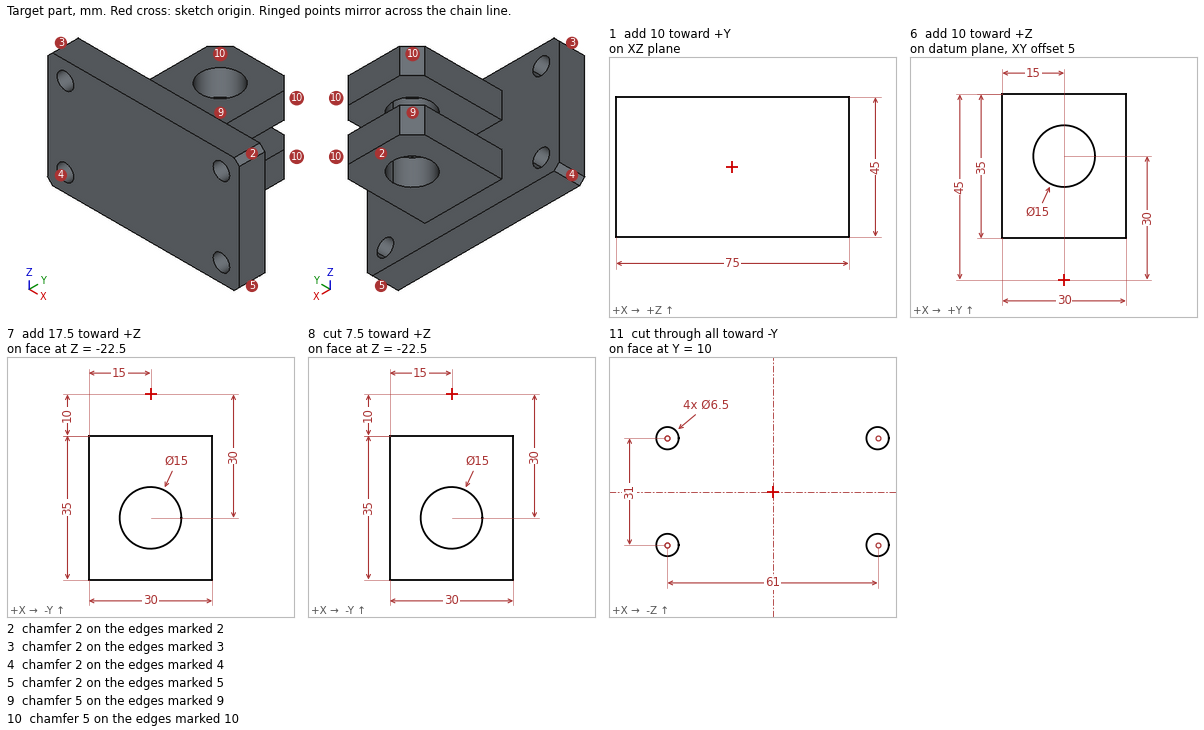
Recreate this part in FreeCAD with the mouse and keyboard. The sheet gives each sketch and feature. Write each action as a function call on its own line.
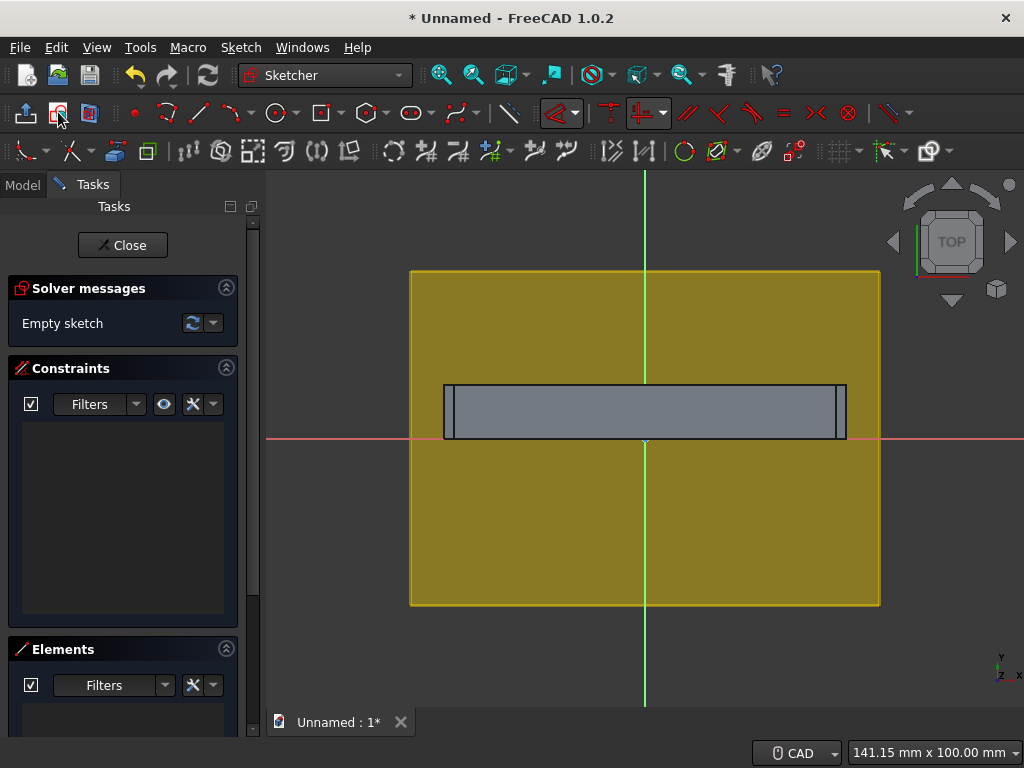
key(q)
key(s)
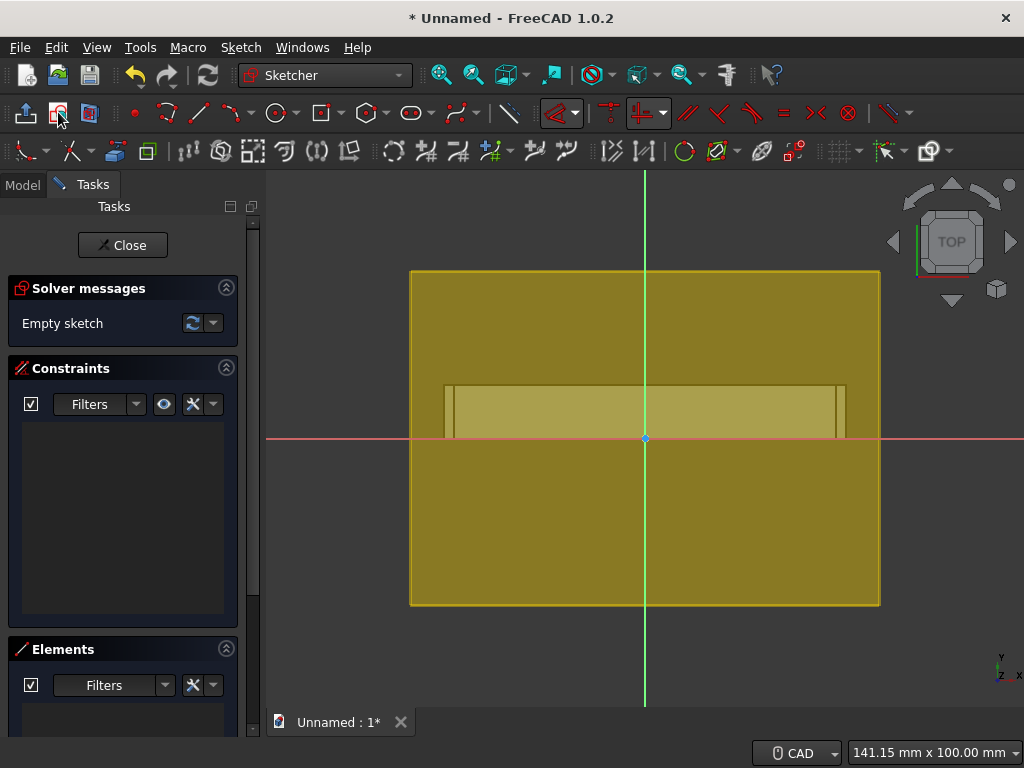
scroll(294, 679, down, 1)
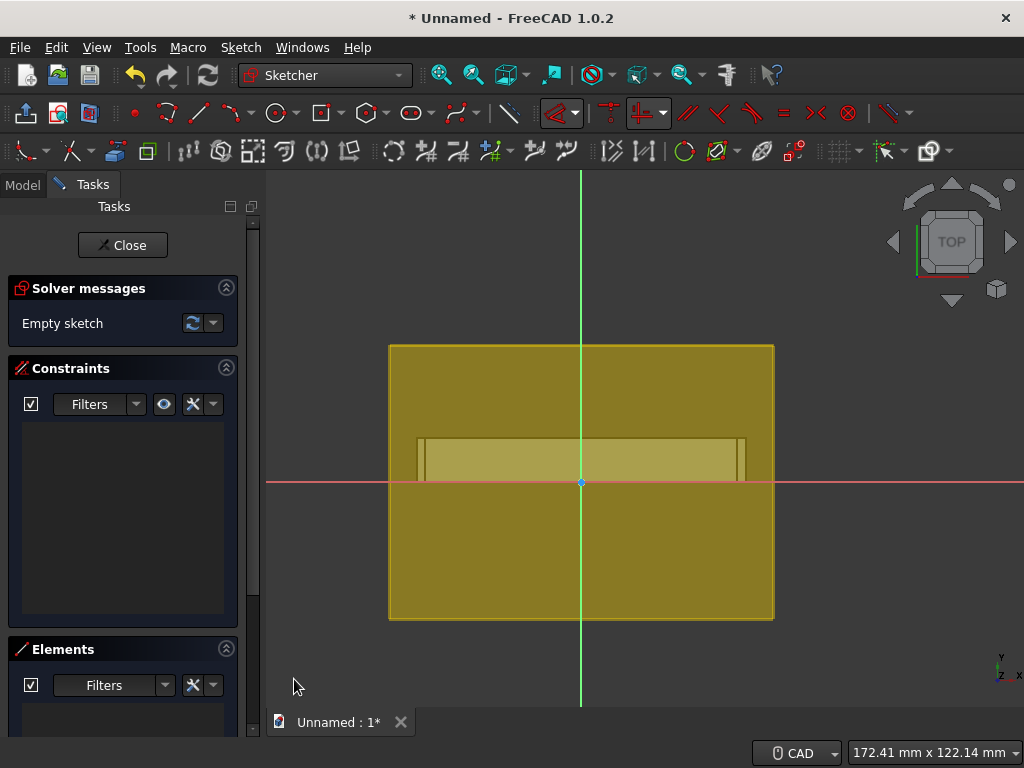
scroll(587, 316, up, 3)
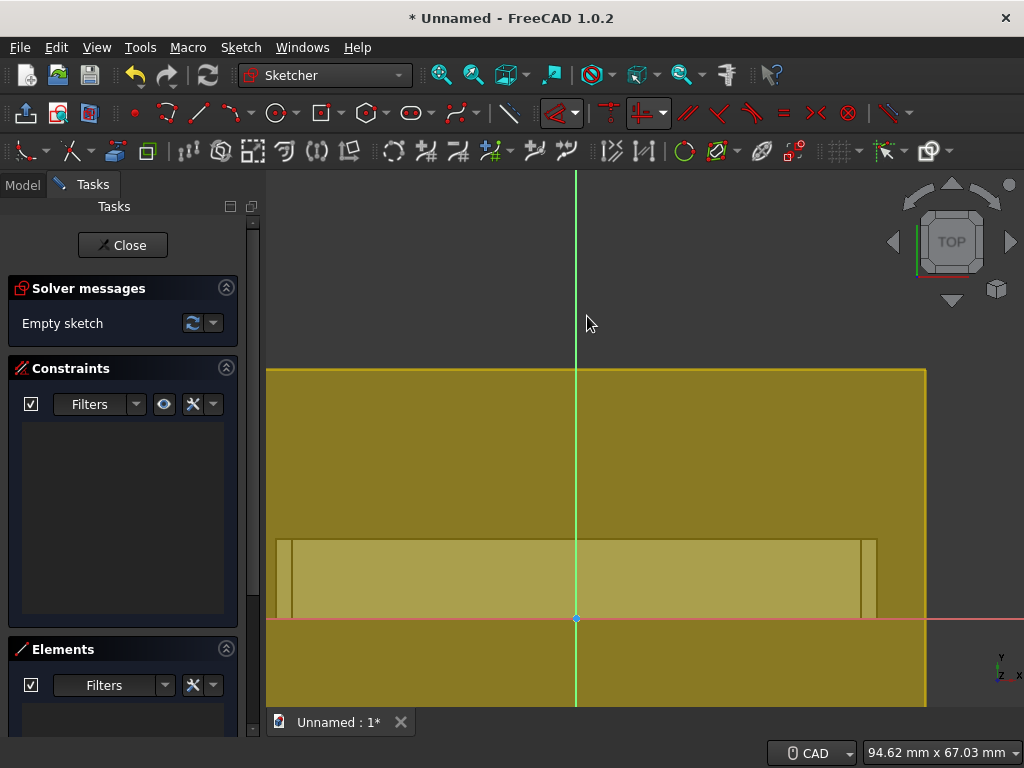
key(g)
key(r)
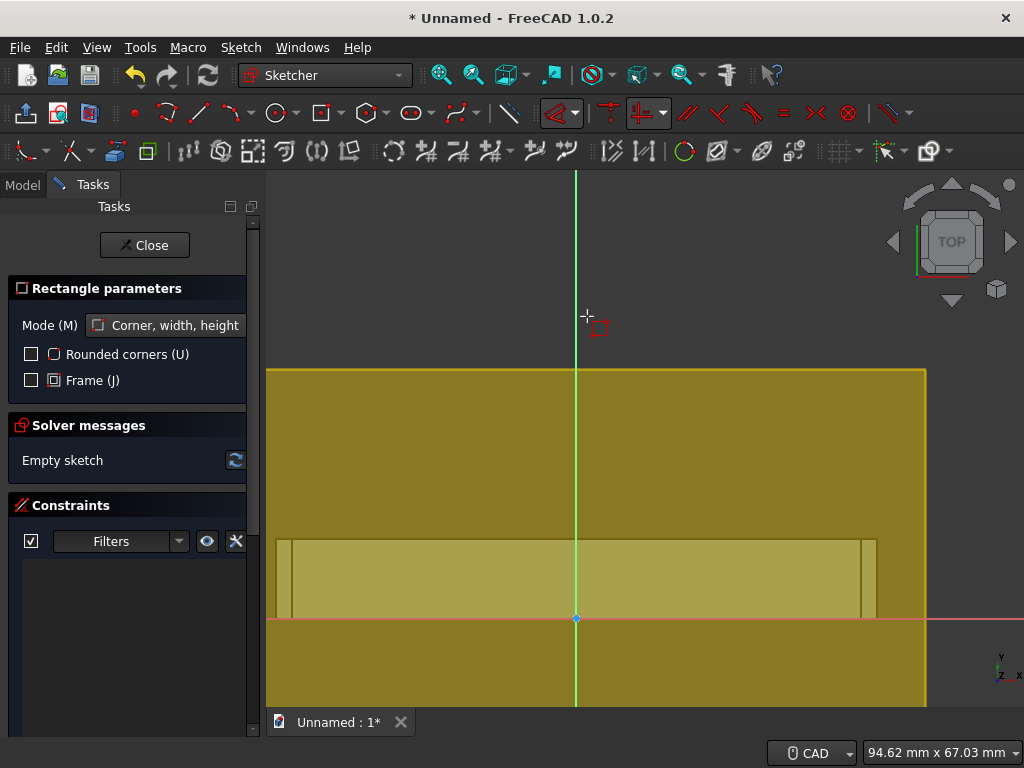
click(456, 258)
click(697, 539)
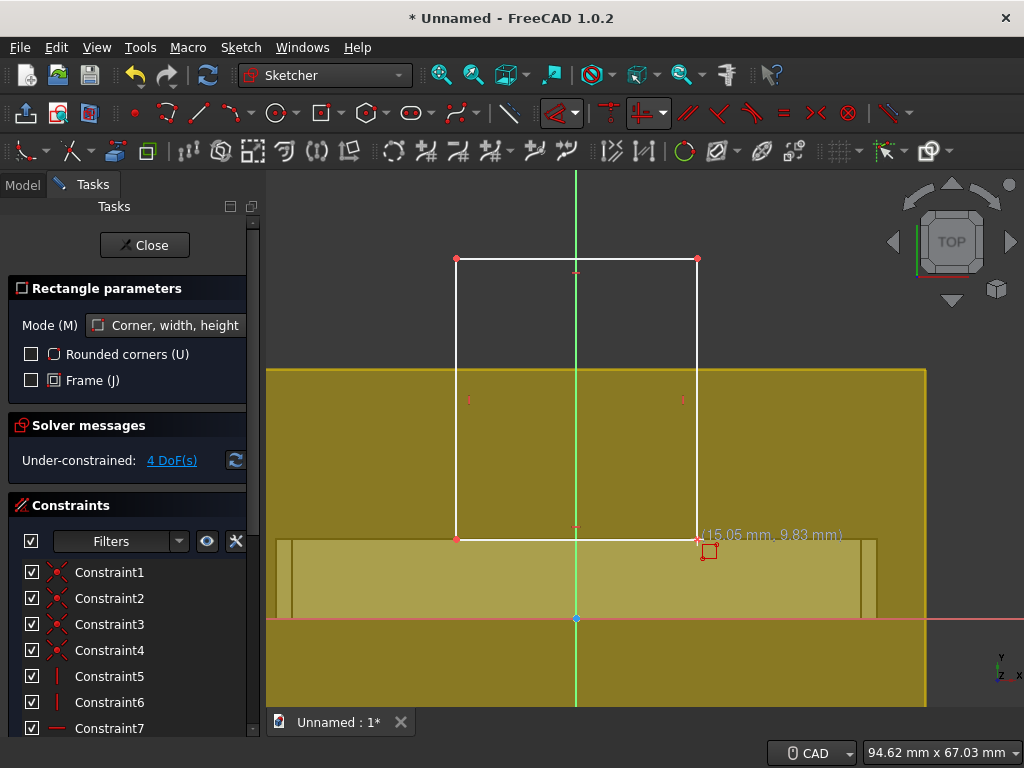
click(276, 114)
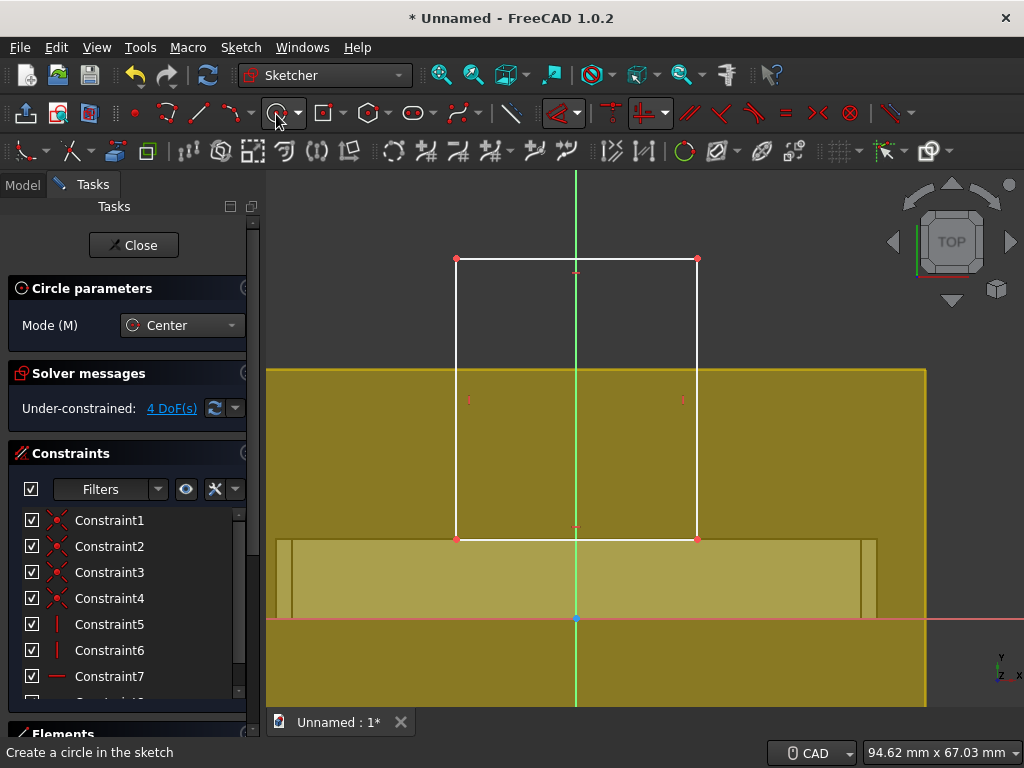
click(576, 378)
click(619, 336)
key(Escape)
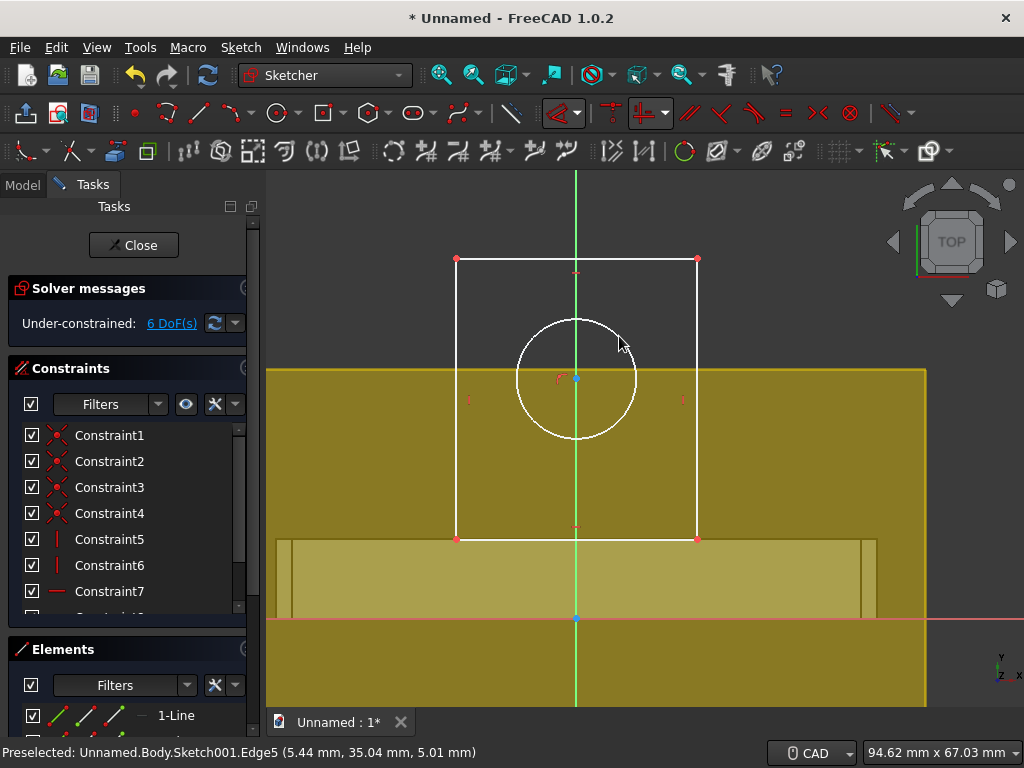
key(d)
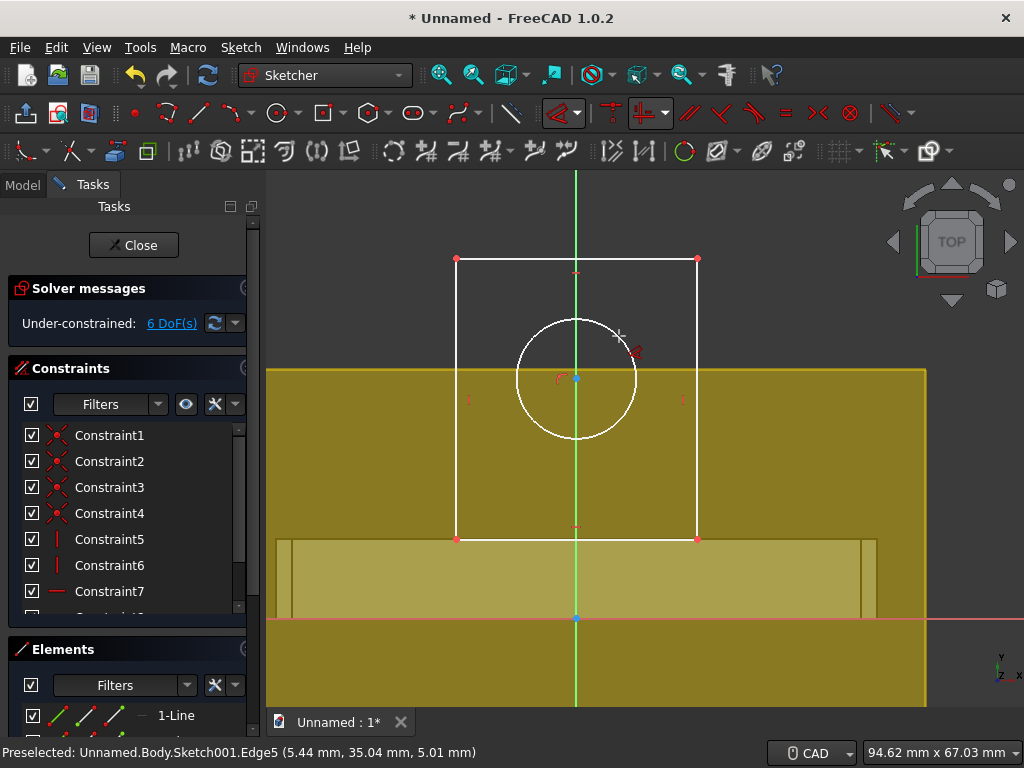
click(619, 337)
click(642, 315)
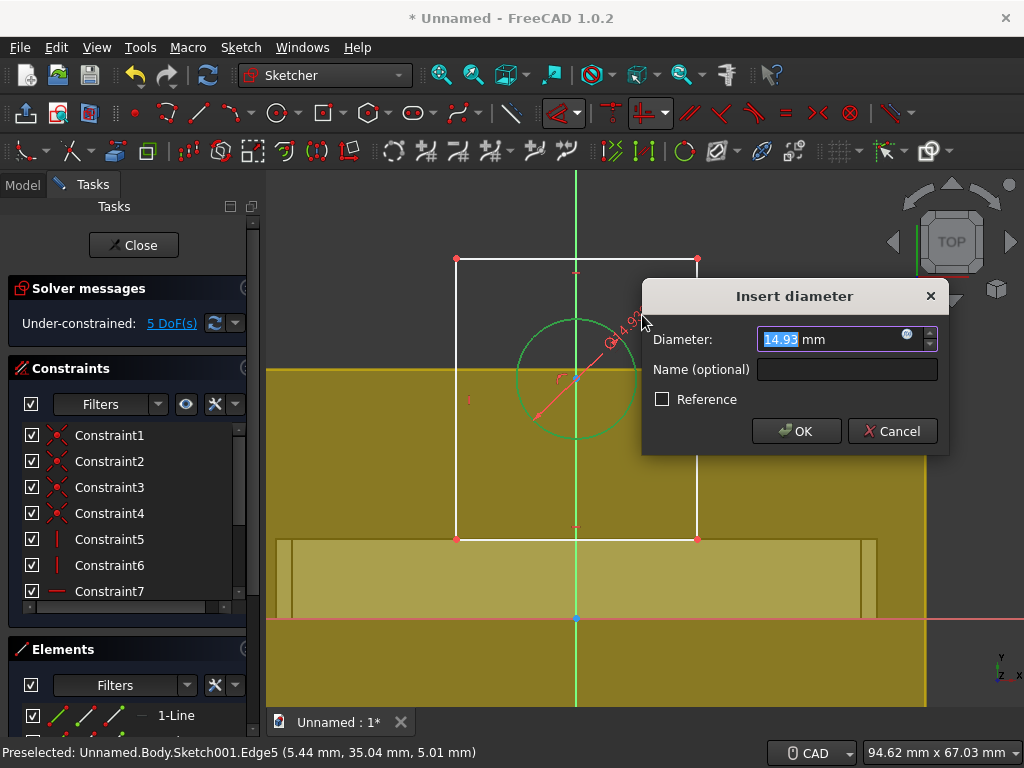
text(15)
key(Return)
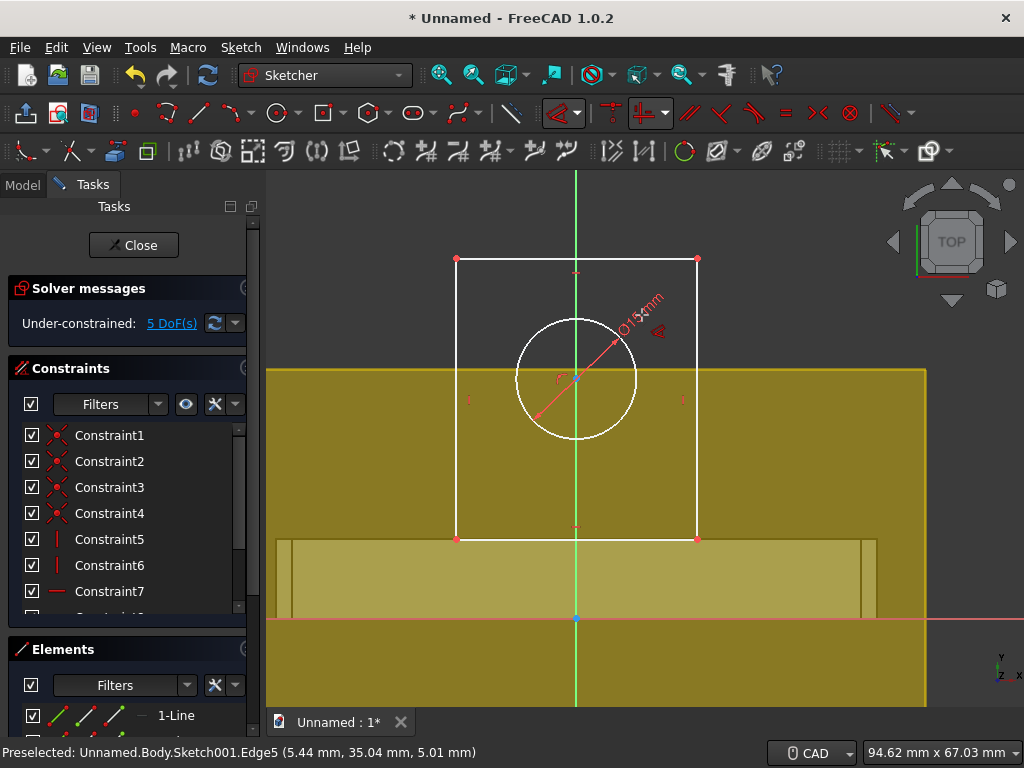
click(456, 343)
click(422, 399)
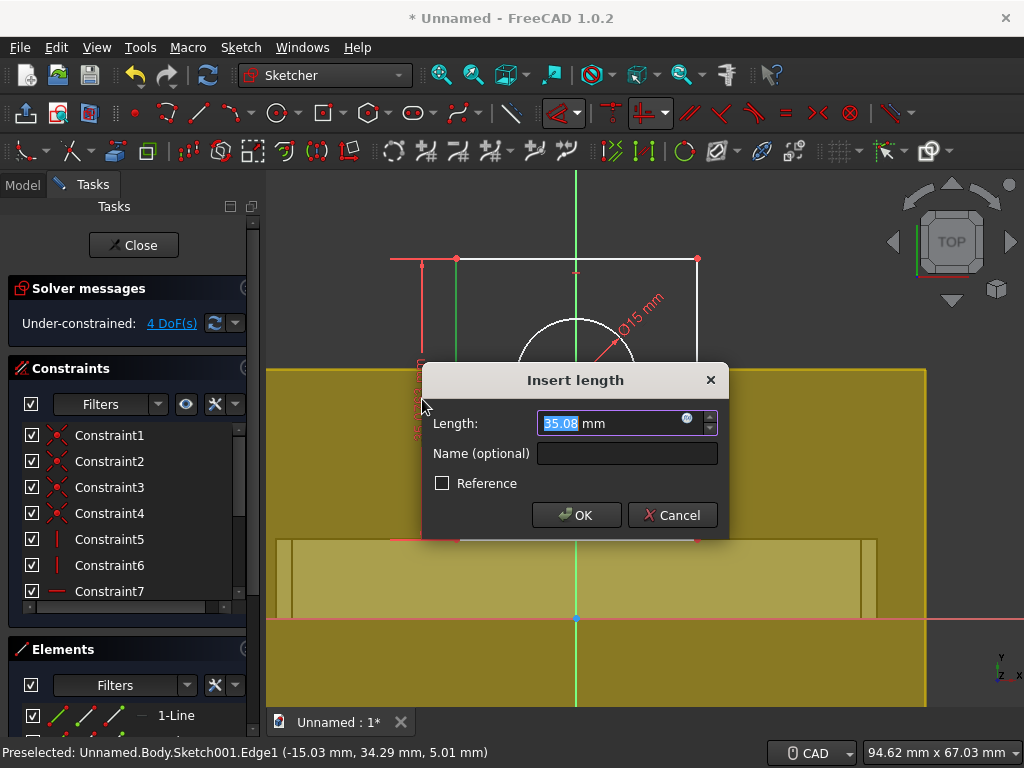
text(35)
key(Return)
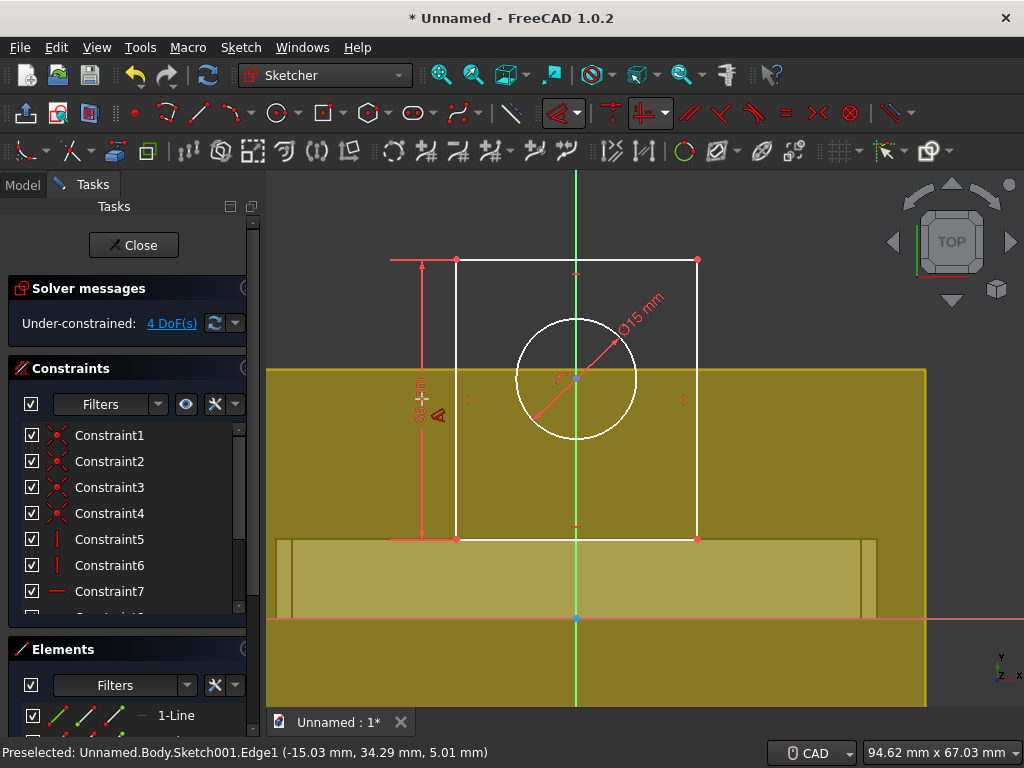
click(528, 540)
click(521, 574)